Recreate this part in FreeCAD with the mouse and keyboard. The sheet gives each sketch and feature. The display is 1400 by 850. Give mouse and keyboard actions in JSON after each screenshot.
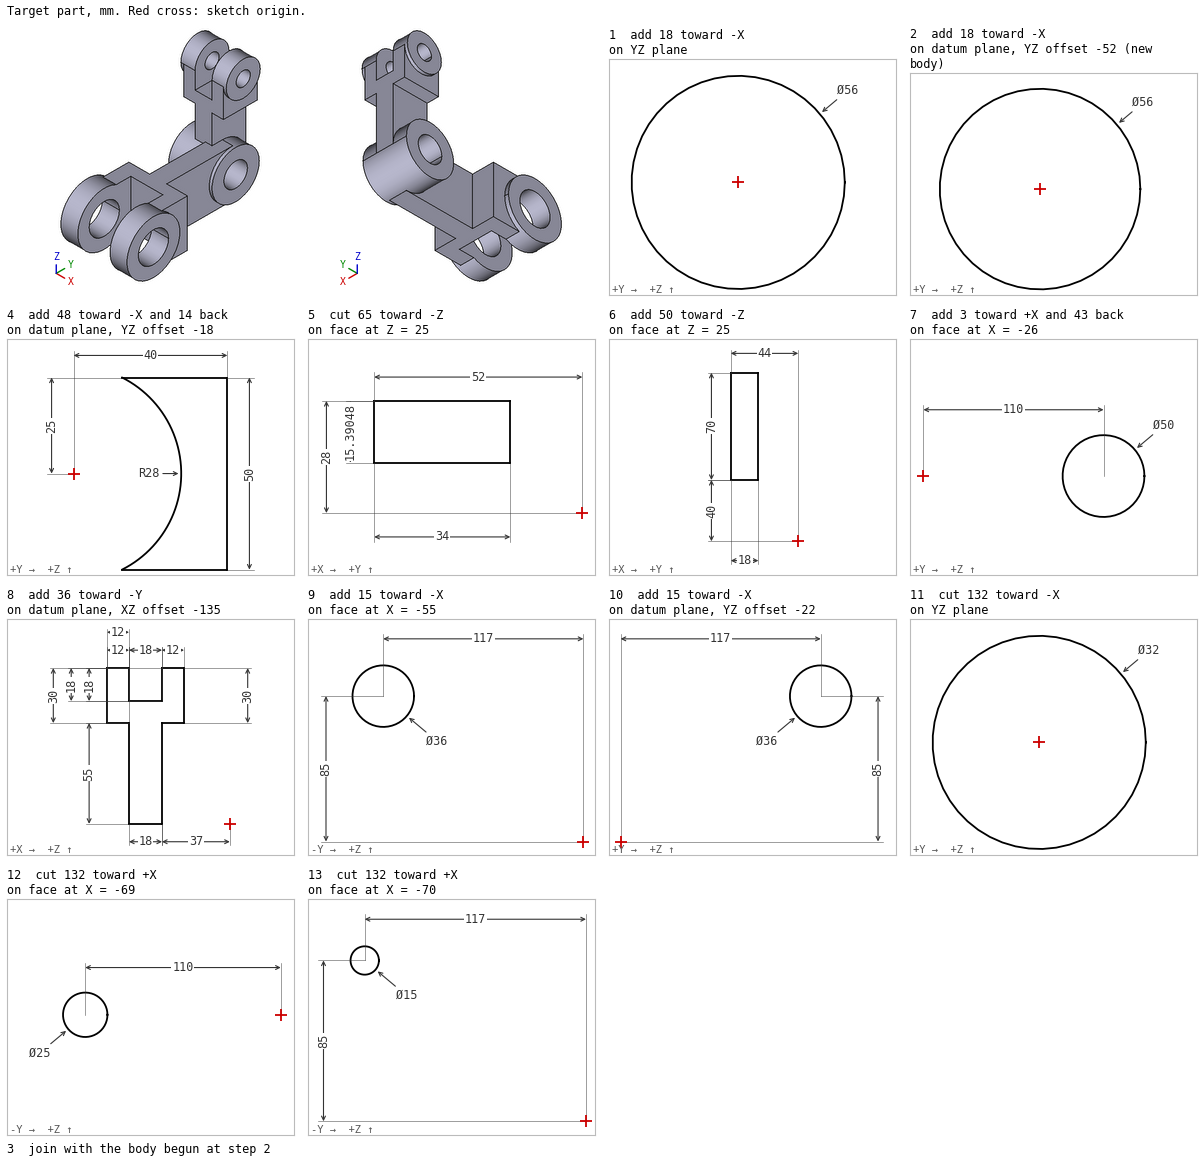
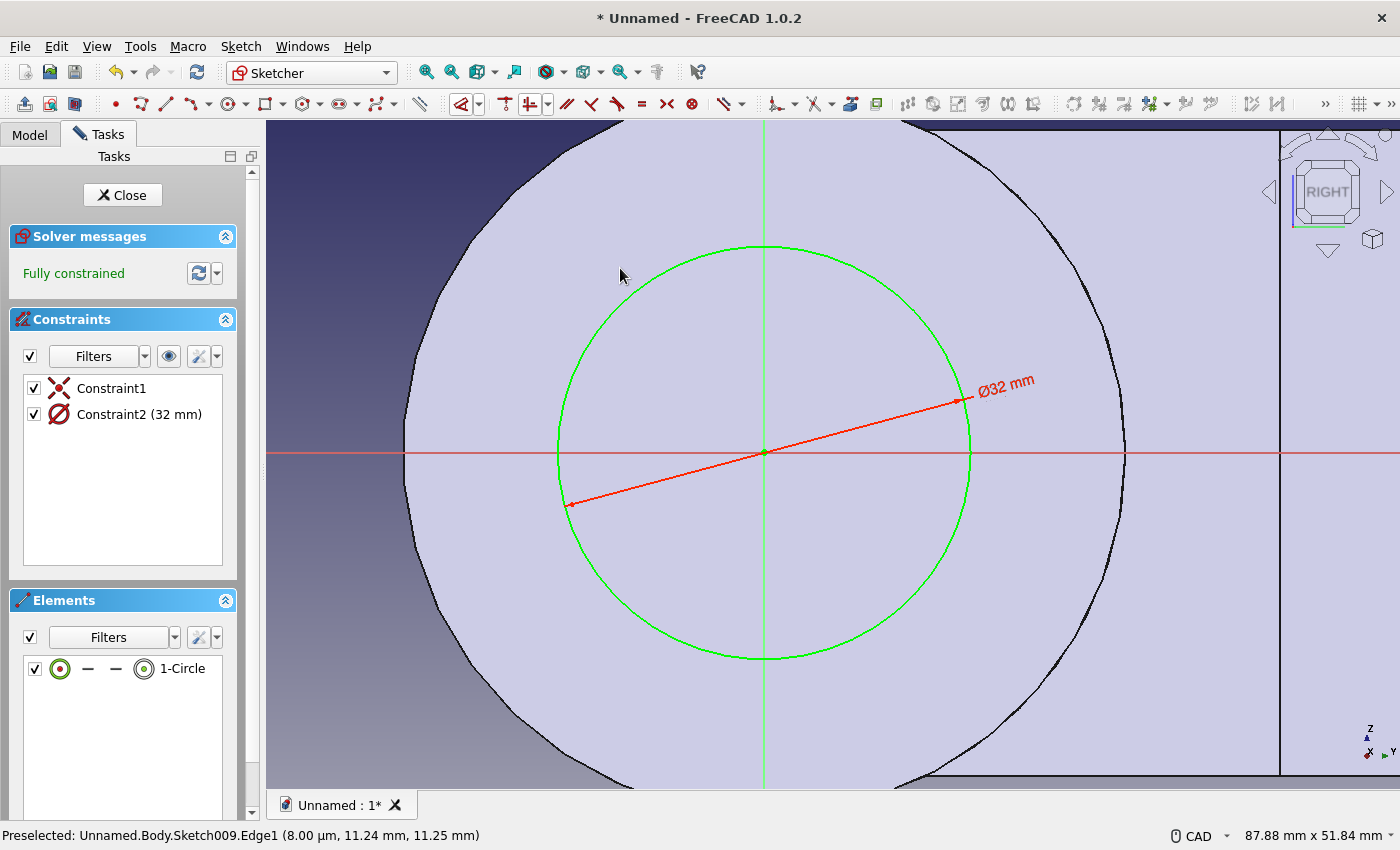
{"action": "left_click", "coordinate": [123, 195]}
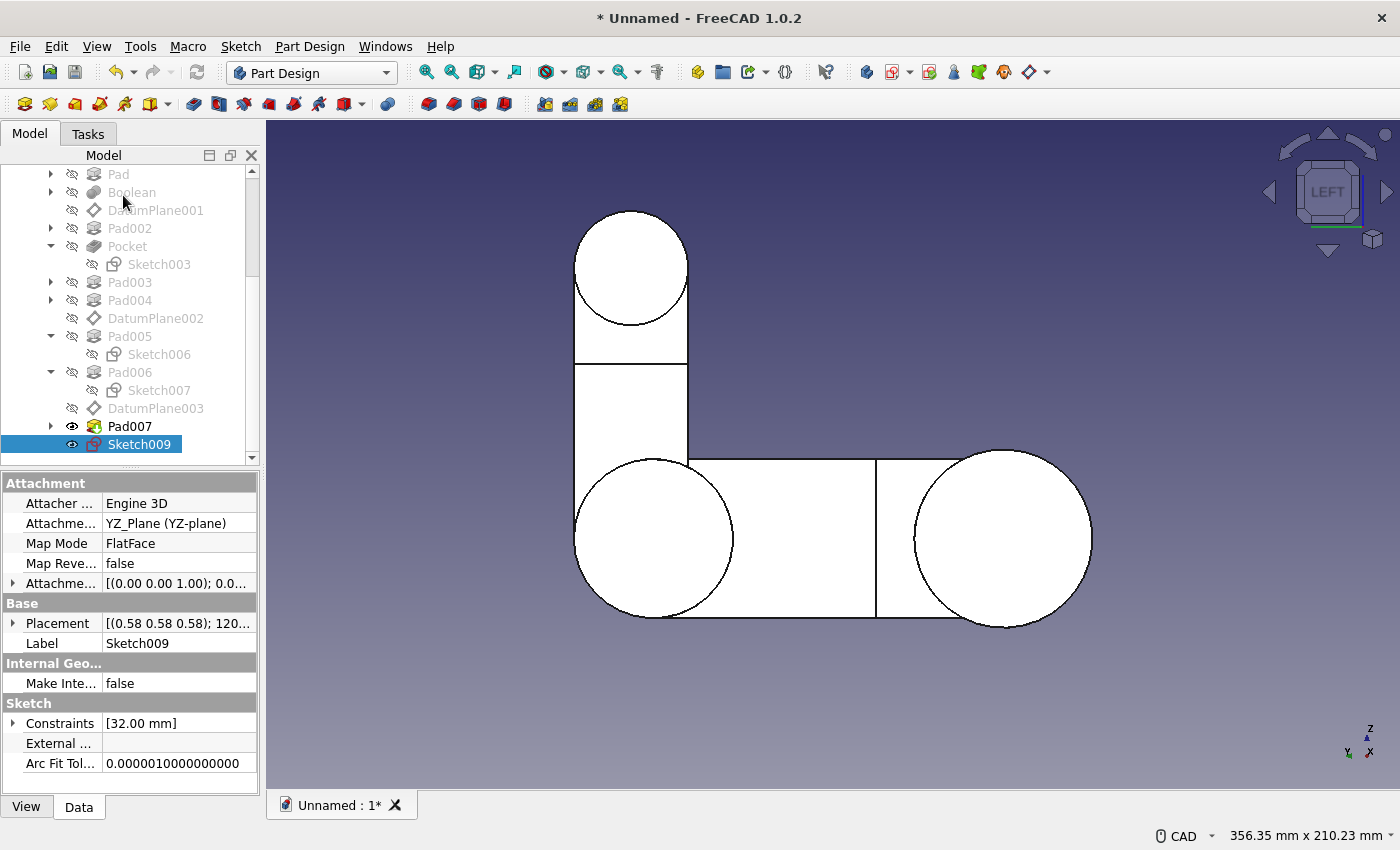
{"action": "left_click", "coordinate": [194, 104]}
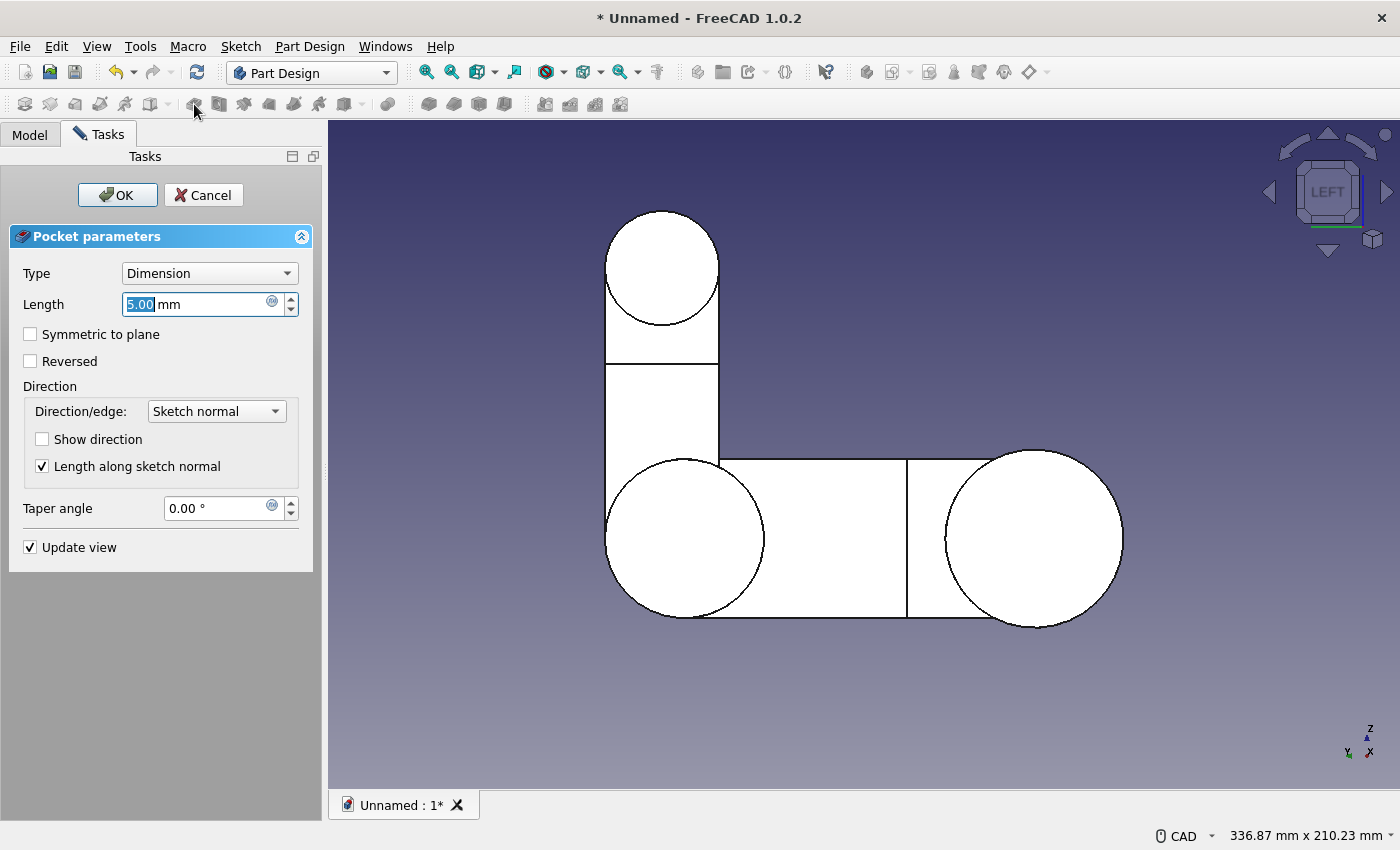
{"action": "type", "text": "132"}
{"action": "key", "text": "Tab"}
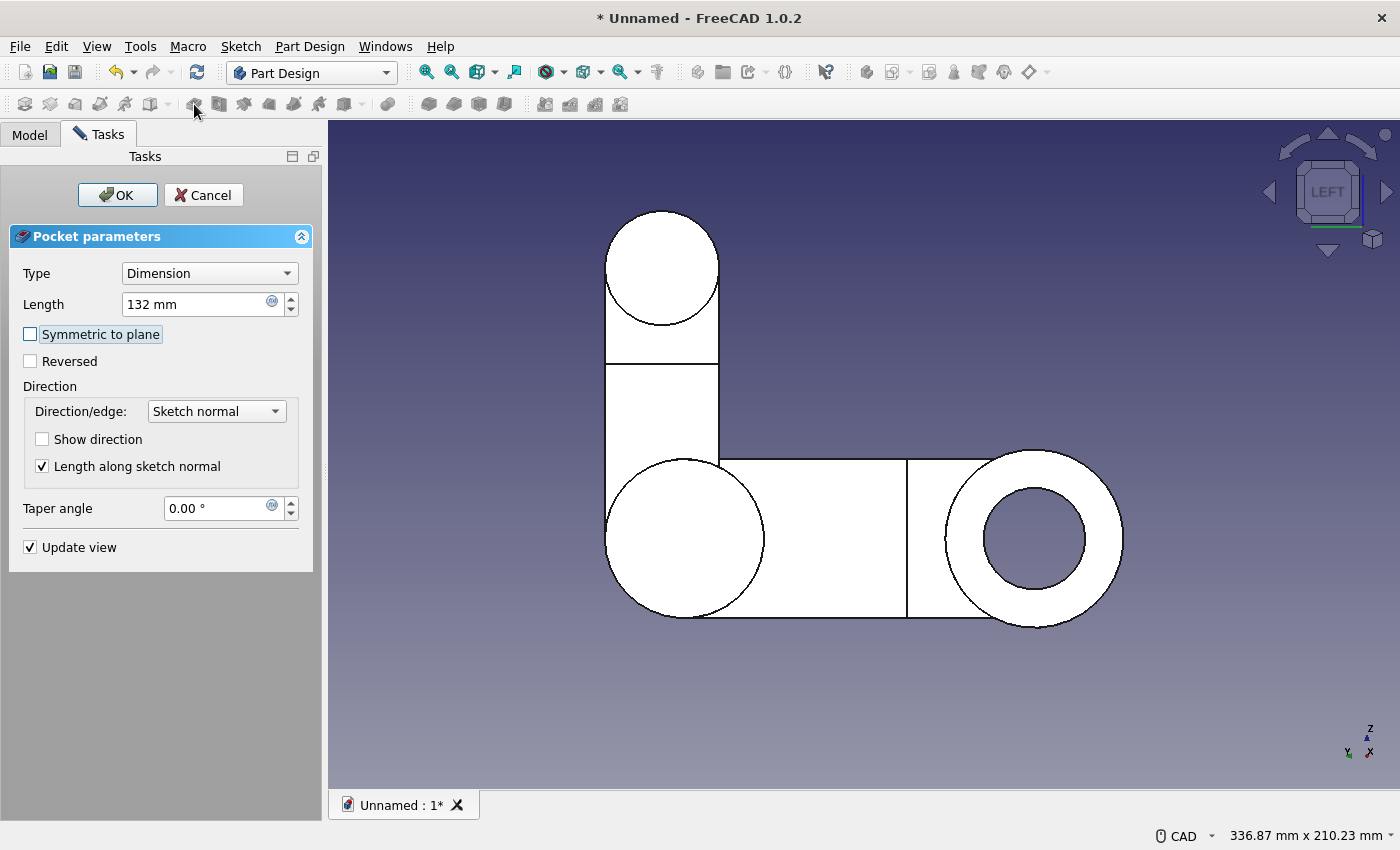
{"action": "left_click", "coordinate": [118, 195]}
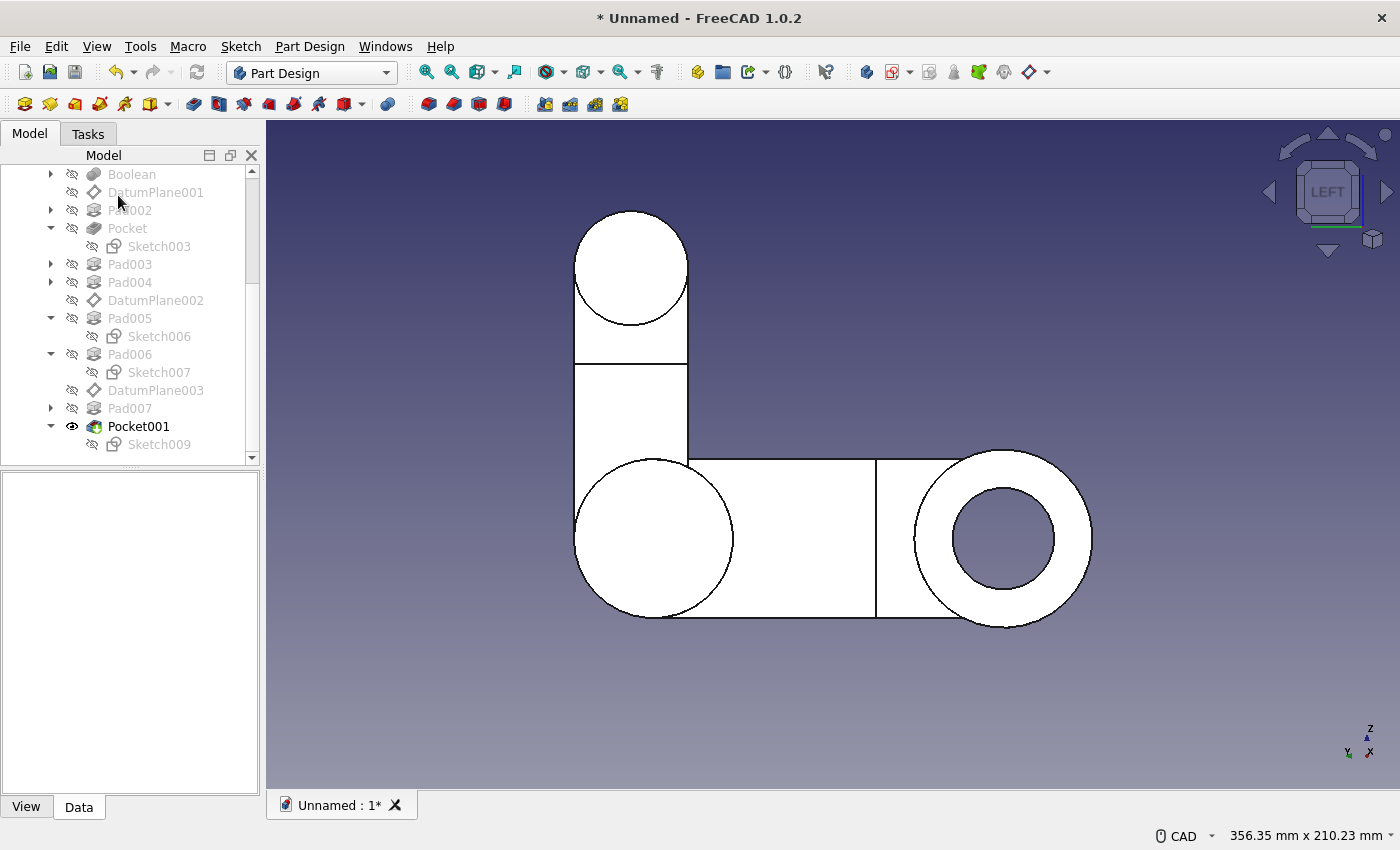
{"action": "left_click", "coordinate": [653, 538]}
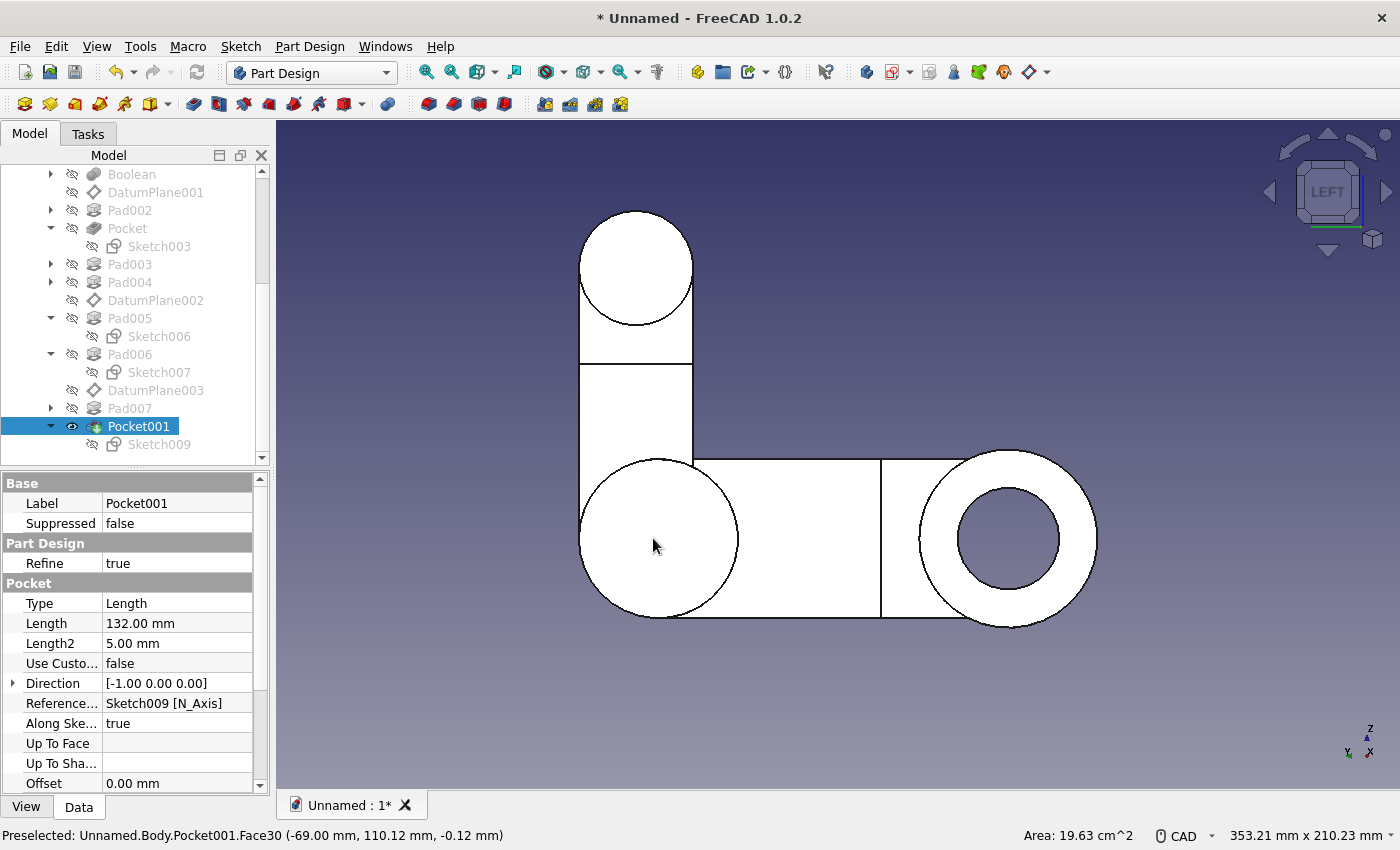
{"action": "left_click", "coordinate": [892, 72]}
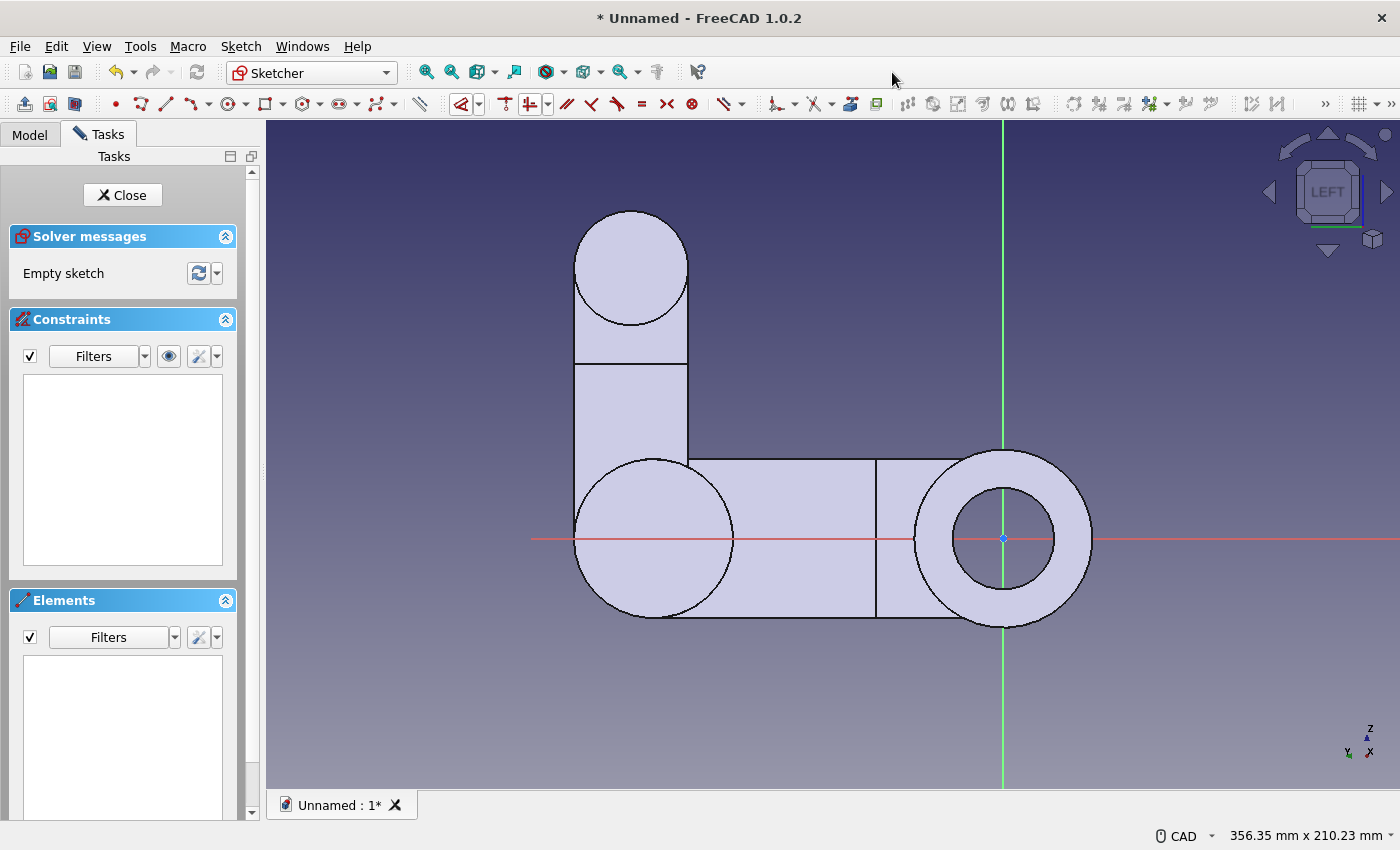
{"action": "left_click", "coordinate": [75, 104]}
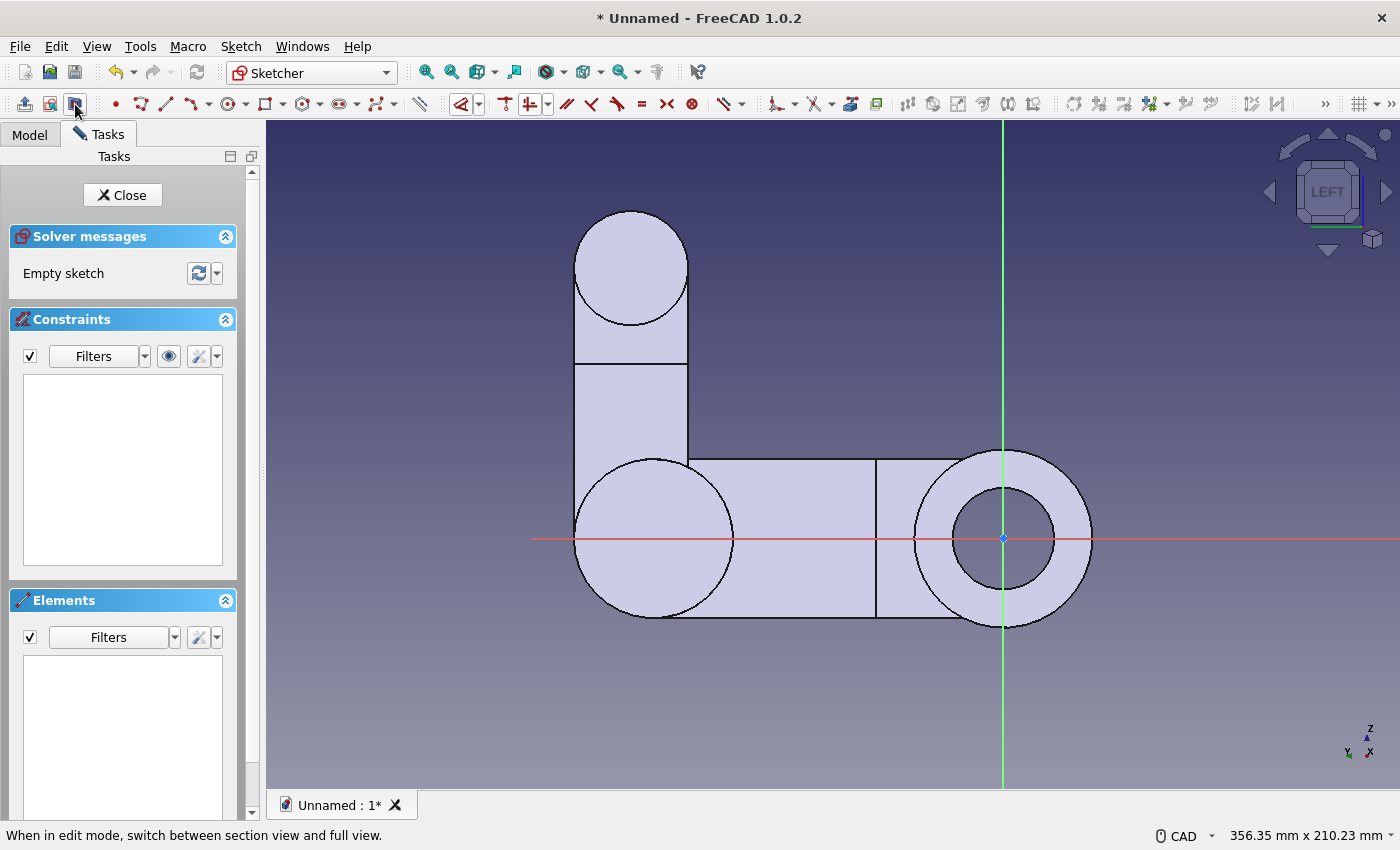
{"action": "scroll", "coordinate": [625, 560], "scroll_direction": "up", "scroll_amount": 8}